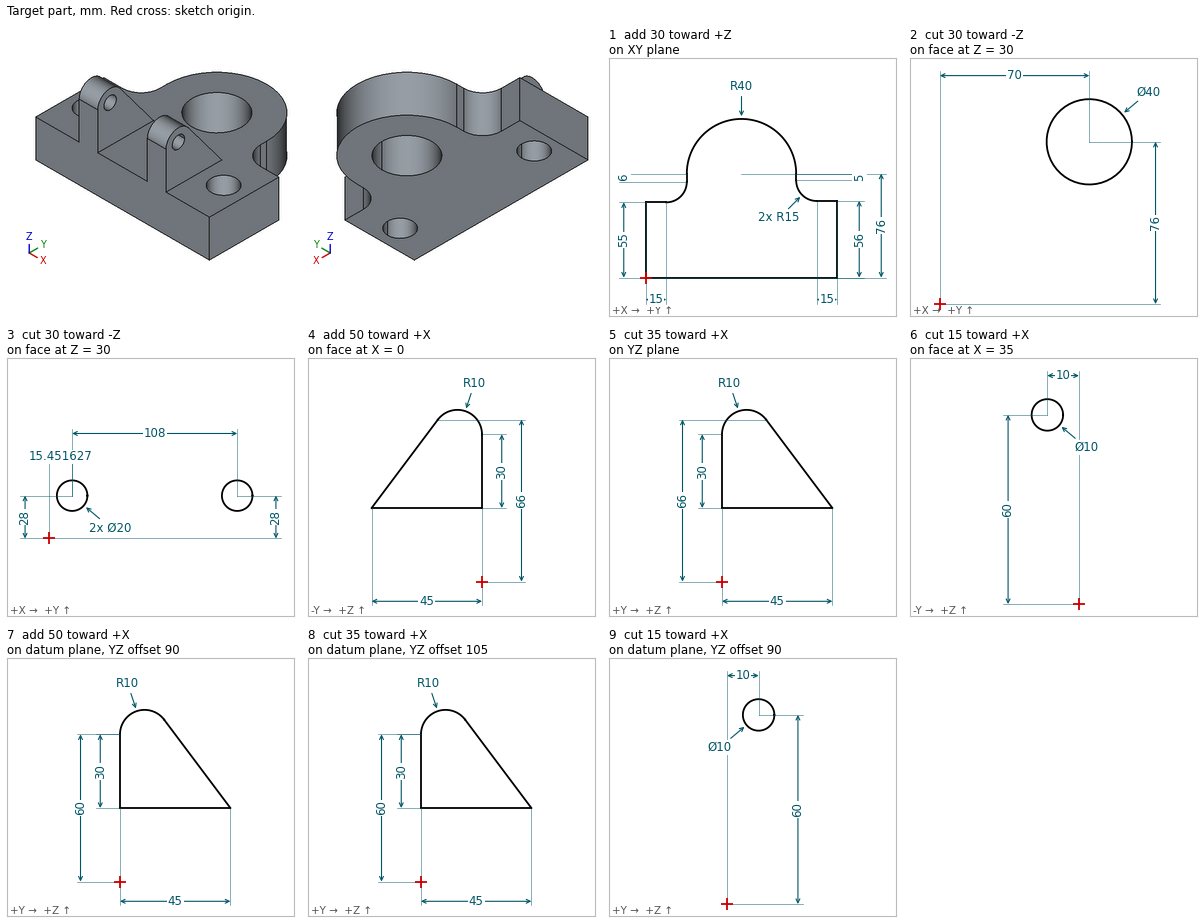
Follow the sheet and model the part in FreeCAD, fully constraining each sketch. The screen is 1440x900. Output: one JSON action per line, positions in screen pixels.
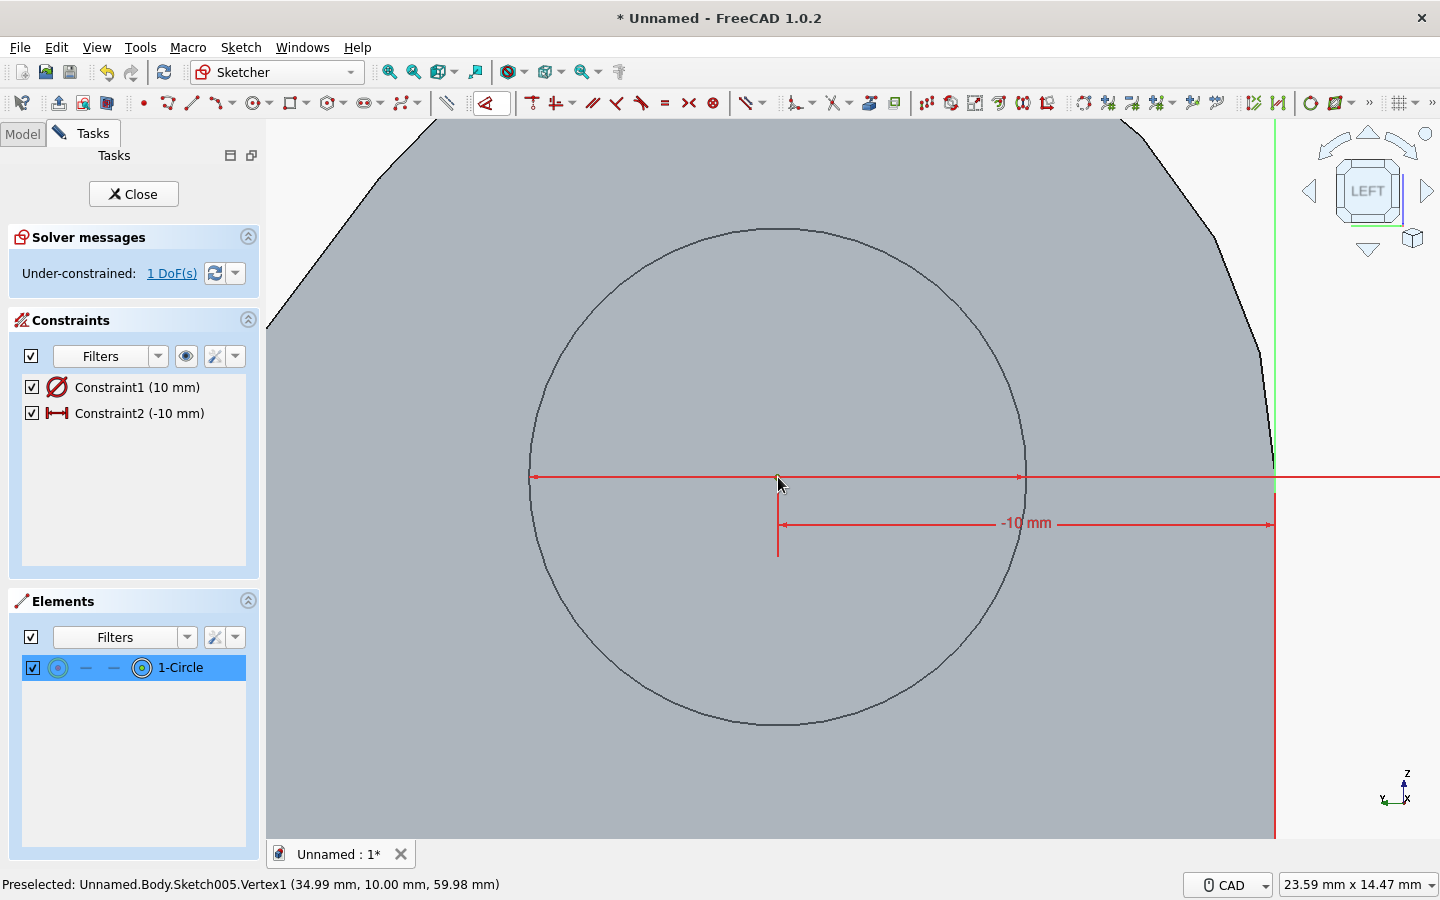
{"action": "key", "text": "i"}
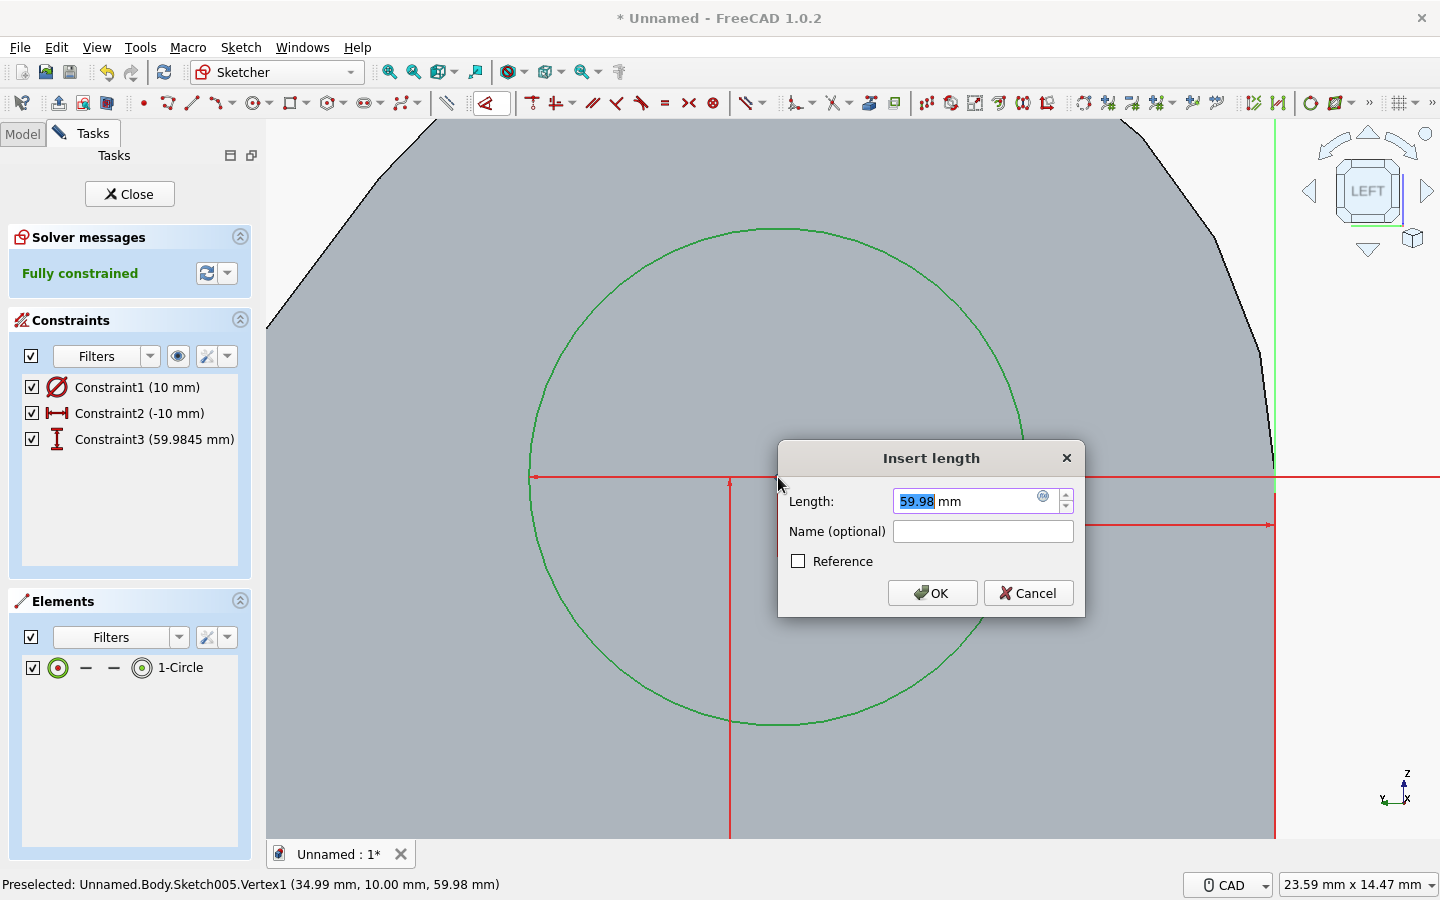
{"action": "type", "text": "60"}
{"action": "key", "text": "Return"}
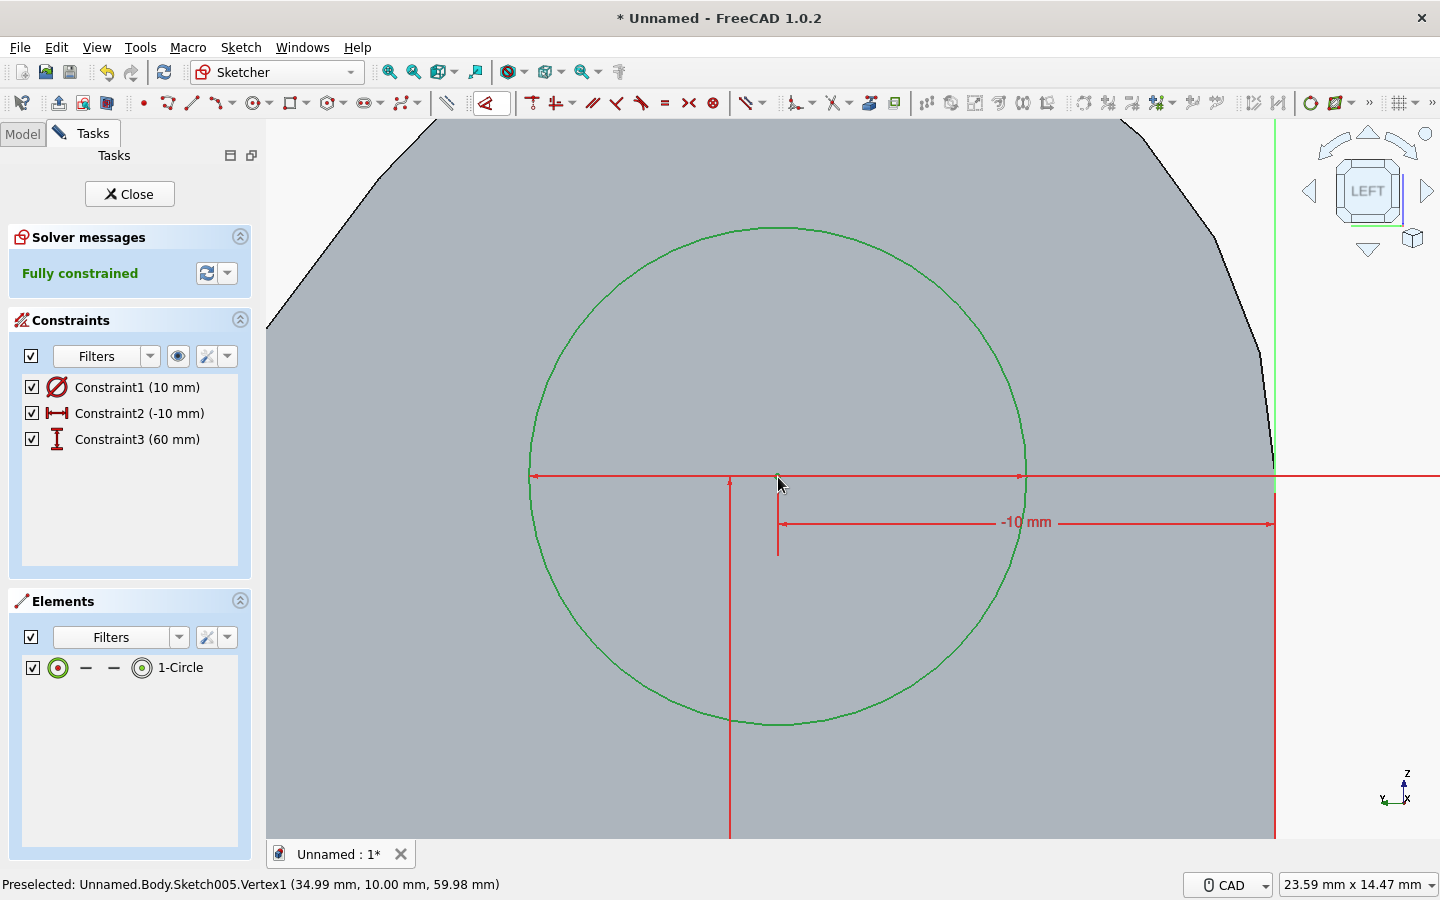
{"action": "left_click", "coordinate": [130, 194]}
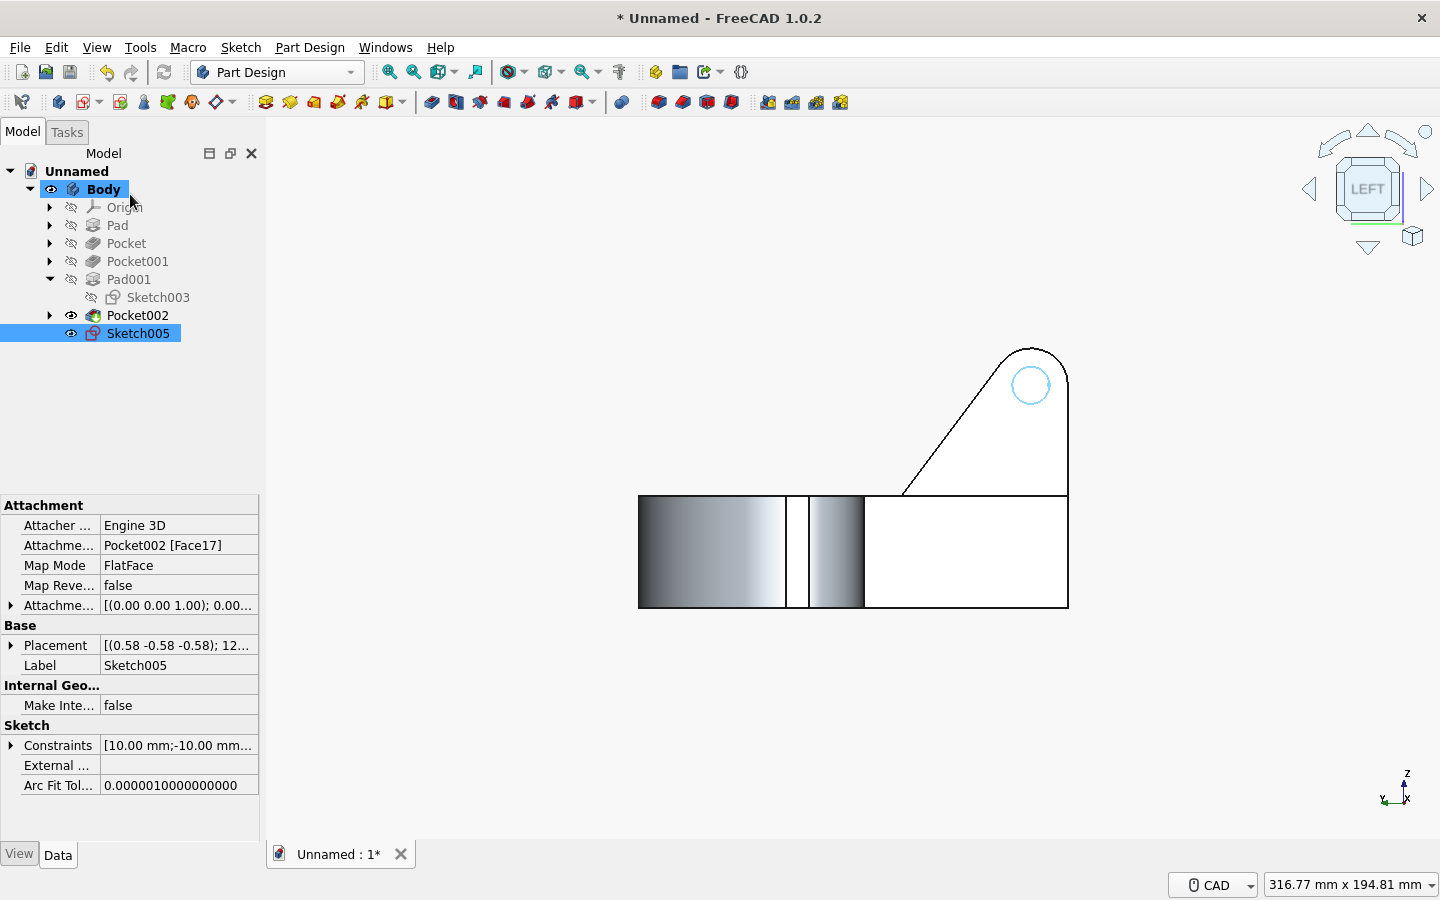
{"action": "left_click", "coordinate": [432, 102]}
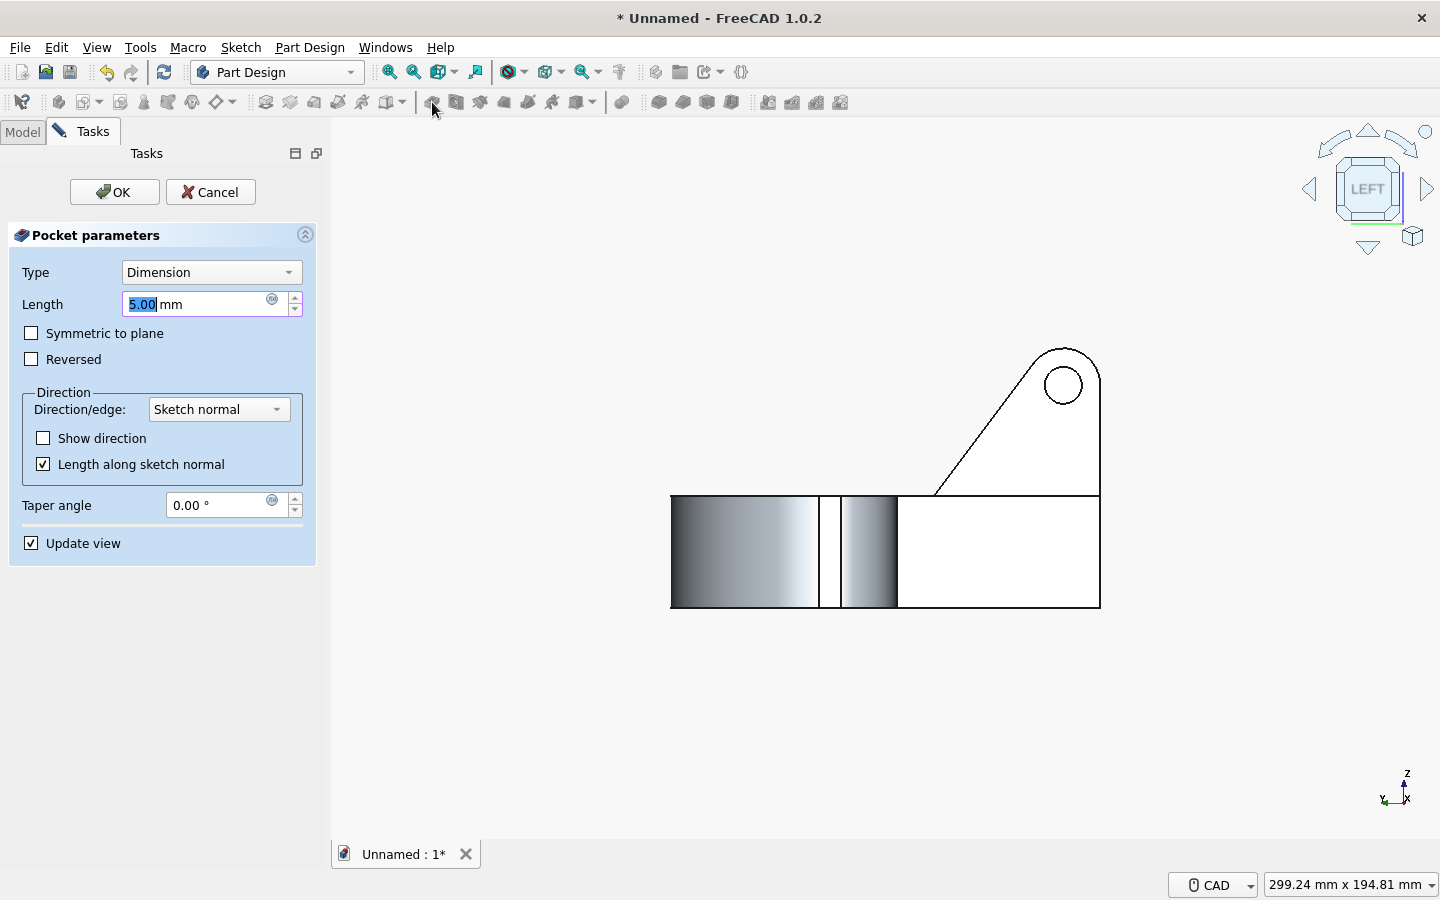
{"action": "type", "text": "15"}
{"action": "key", "text": "Tab"}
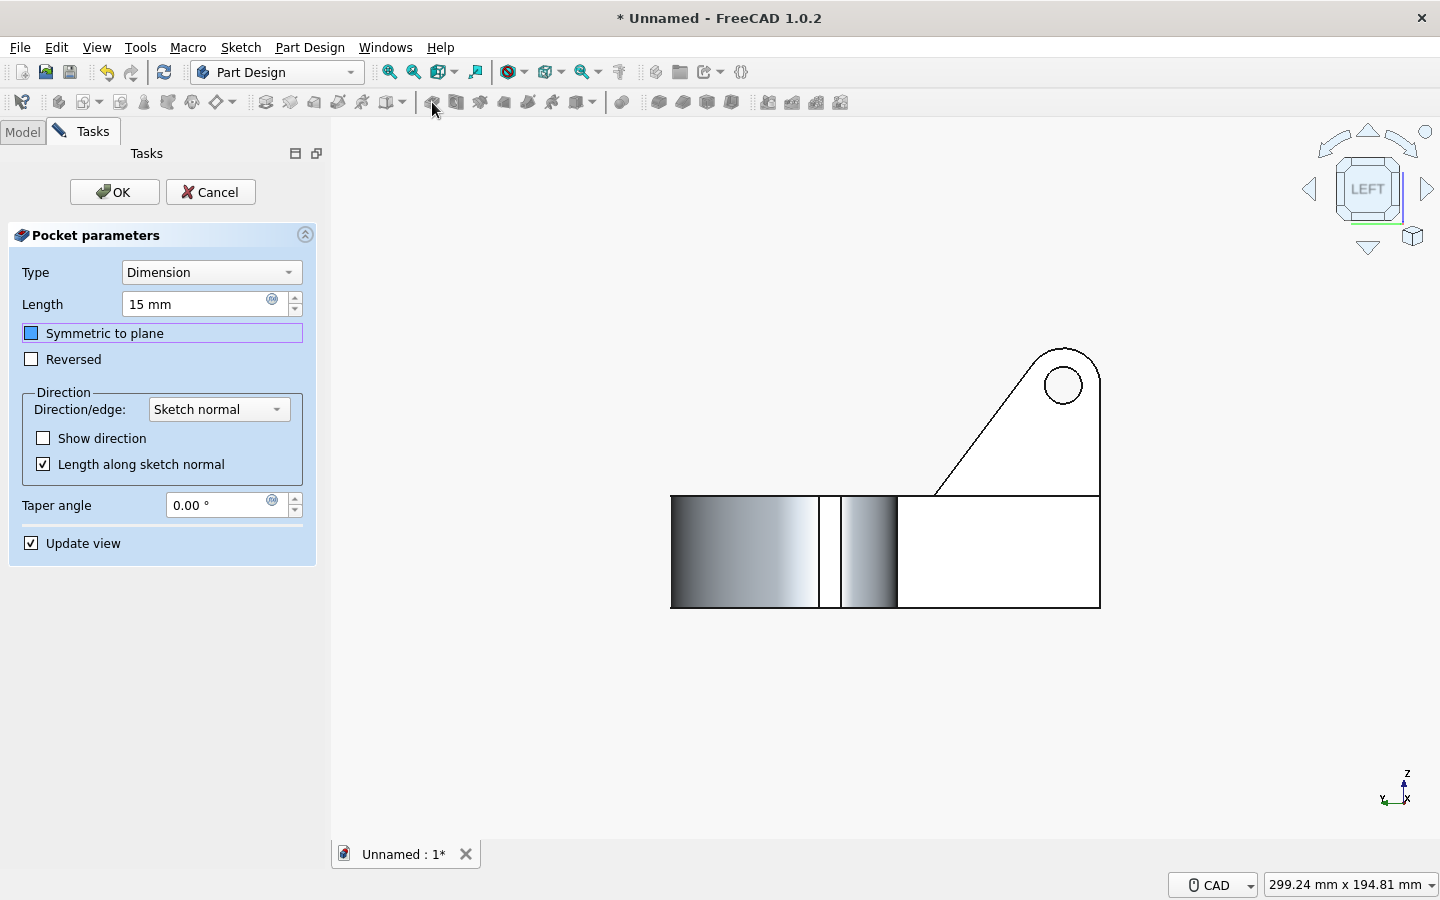
{"action": "left_click", "coordinate": [115, 192]}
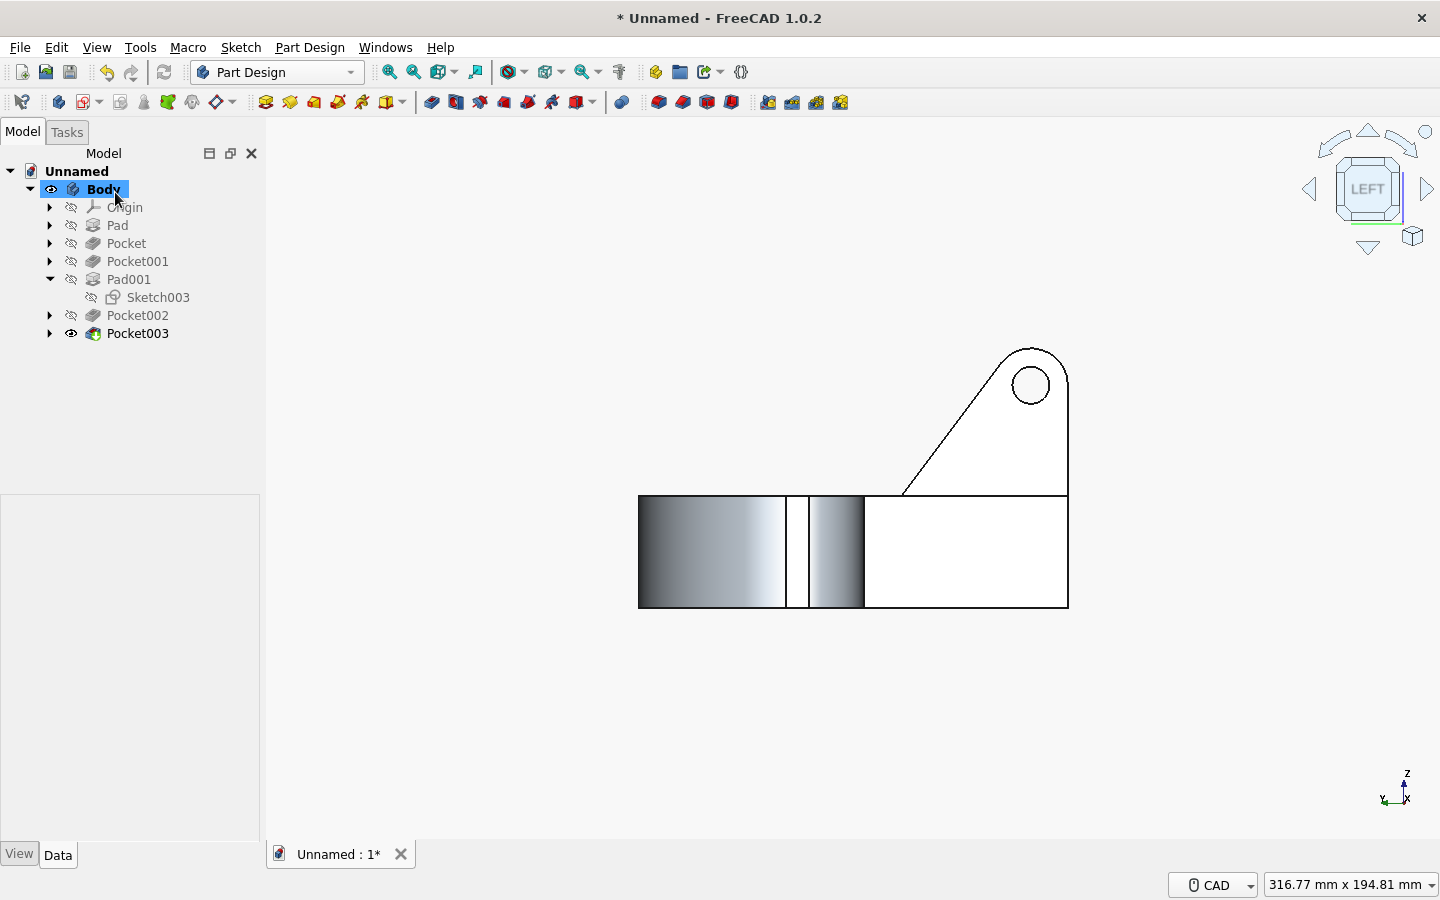
{"action": "key", "text": "v f"}